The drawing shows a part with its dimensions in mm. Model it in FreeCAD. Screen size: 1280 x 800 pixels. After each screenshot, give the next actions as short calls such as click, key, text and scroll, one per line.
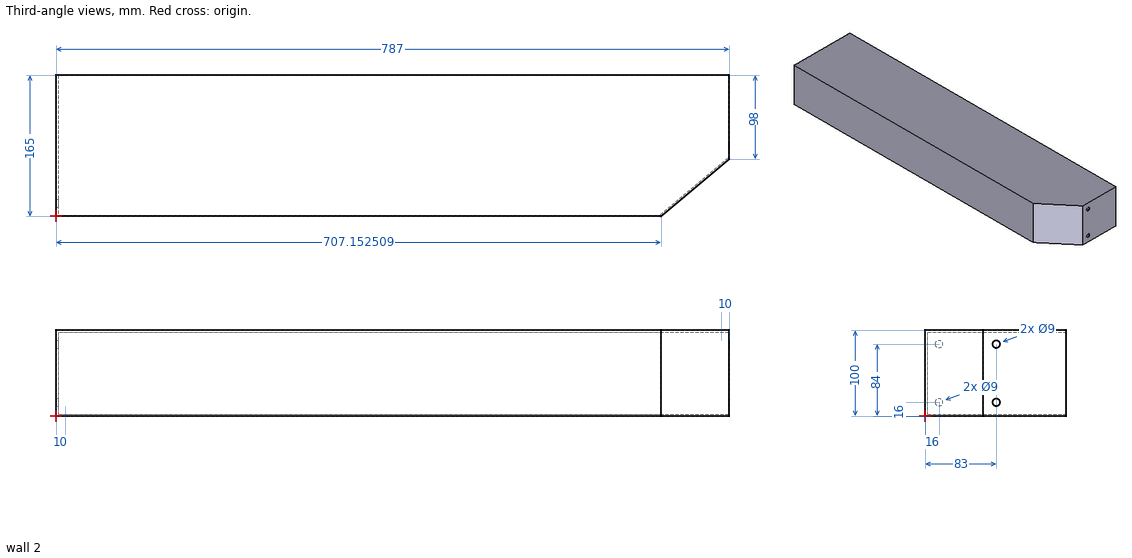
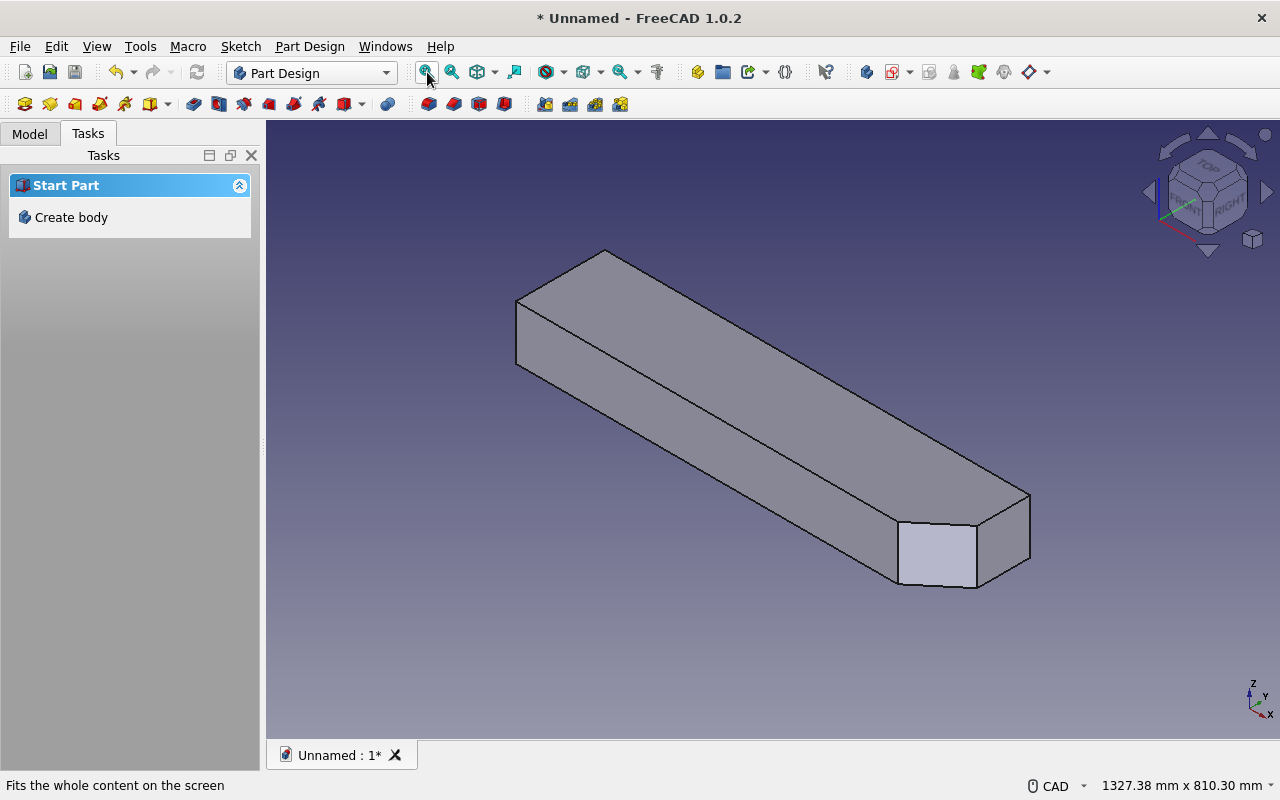
key(2)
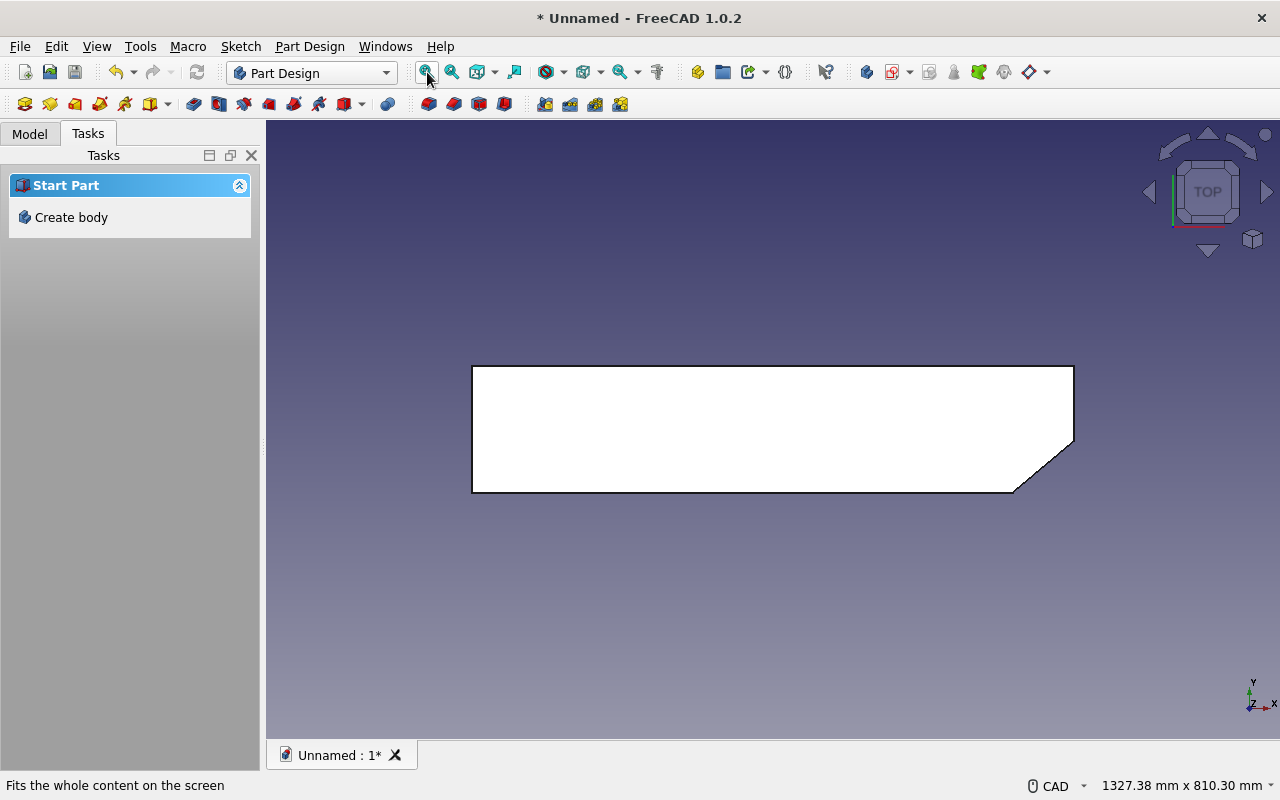
key(1)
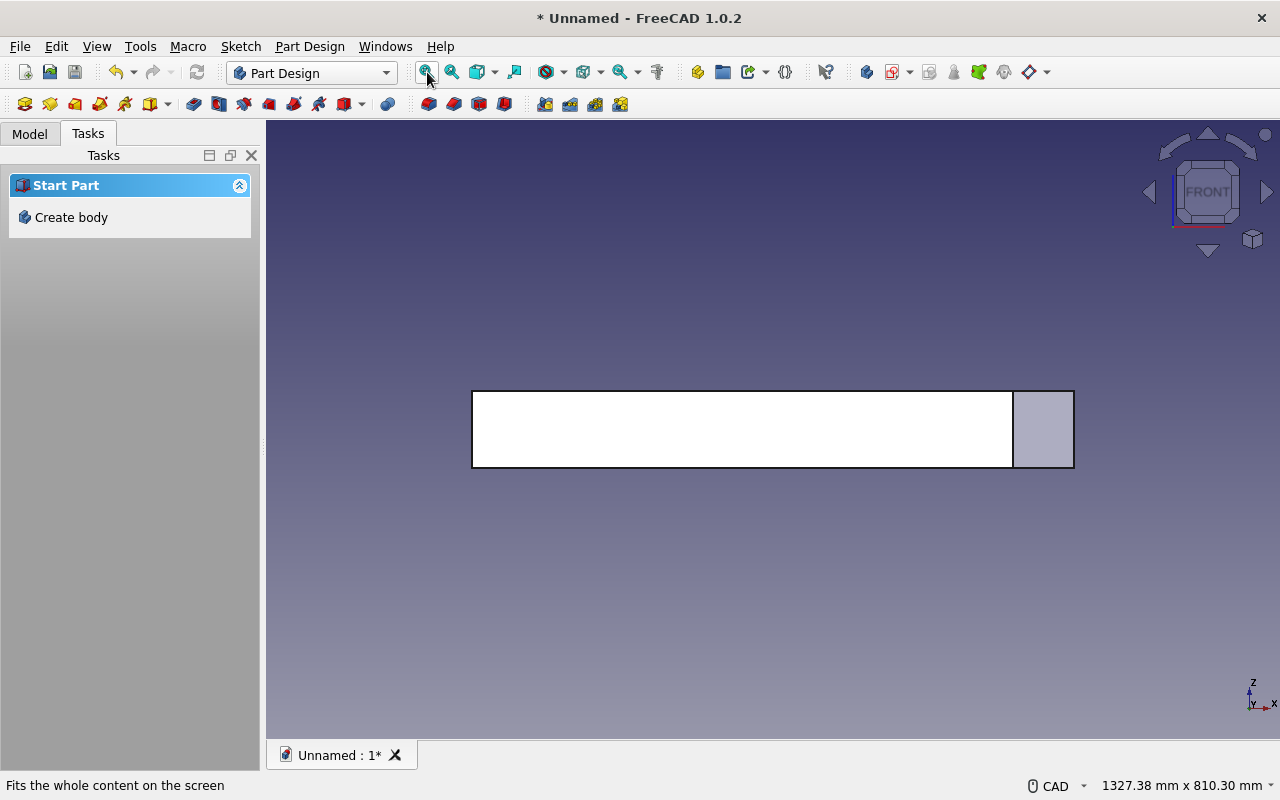
key(3)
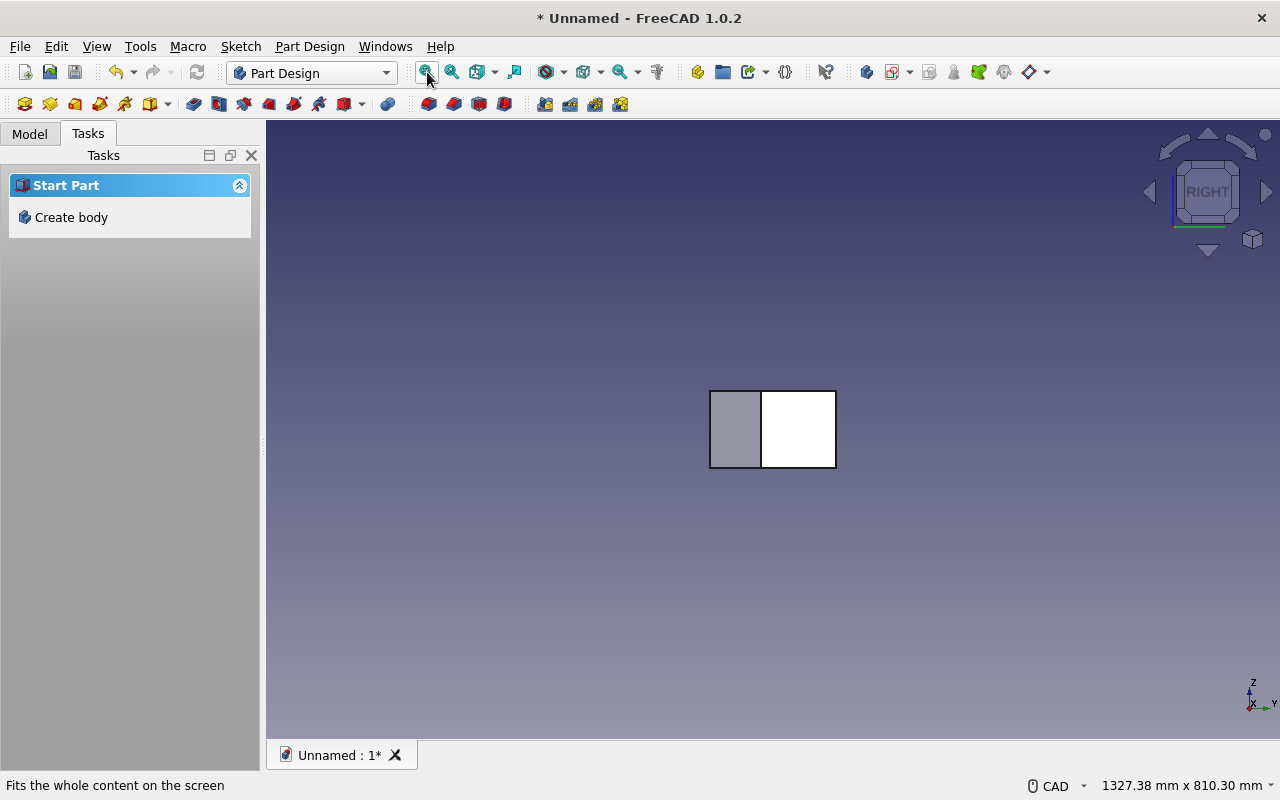
click(427, 72)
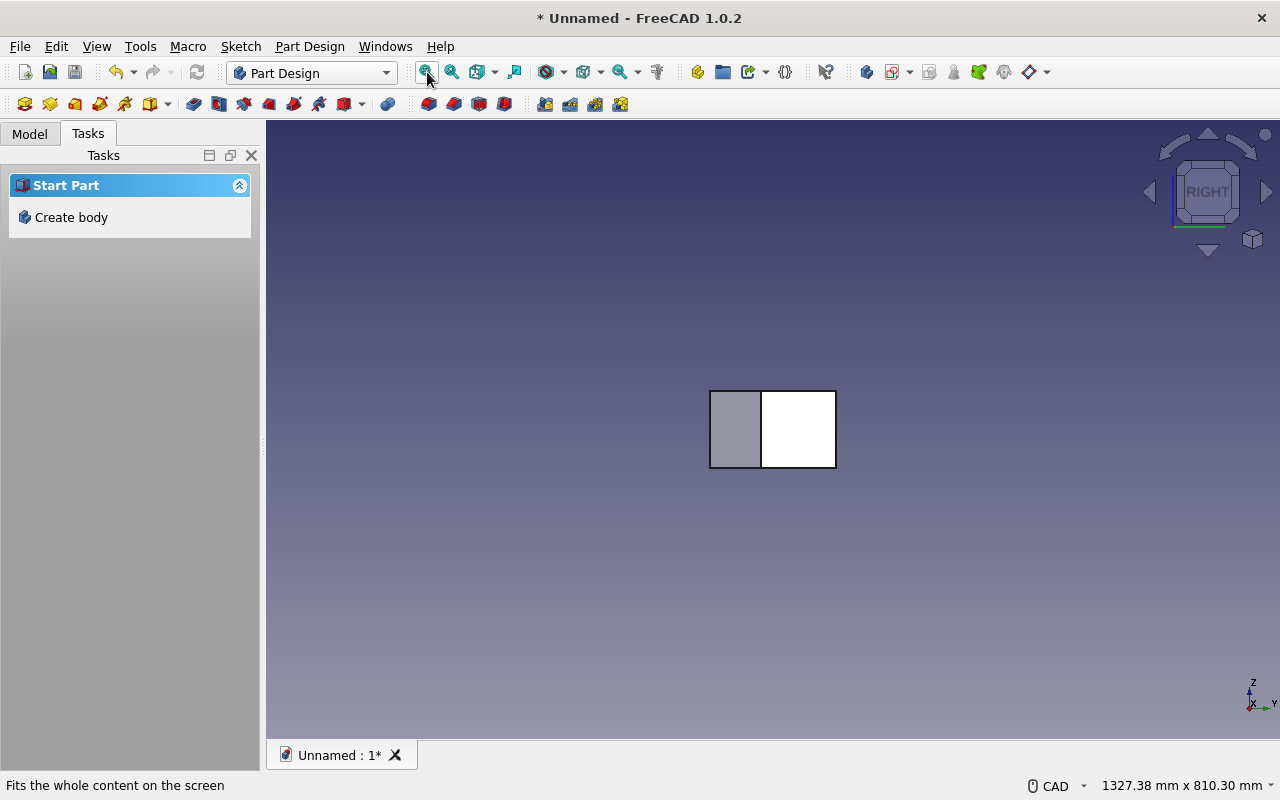
key(5)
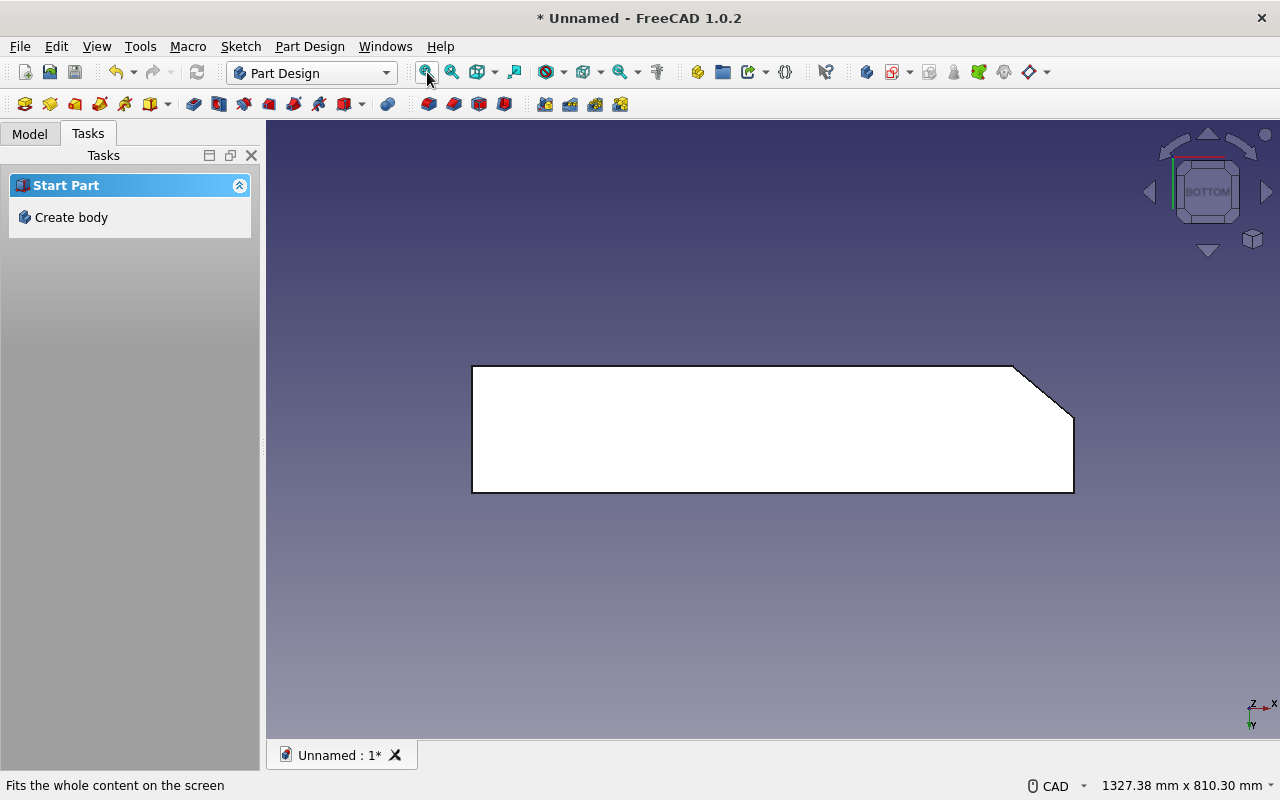
key(4)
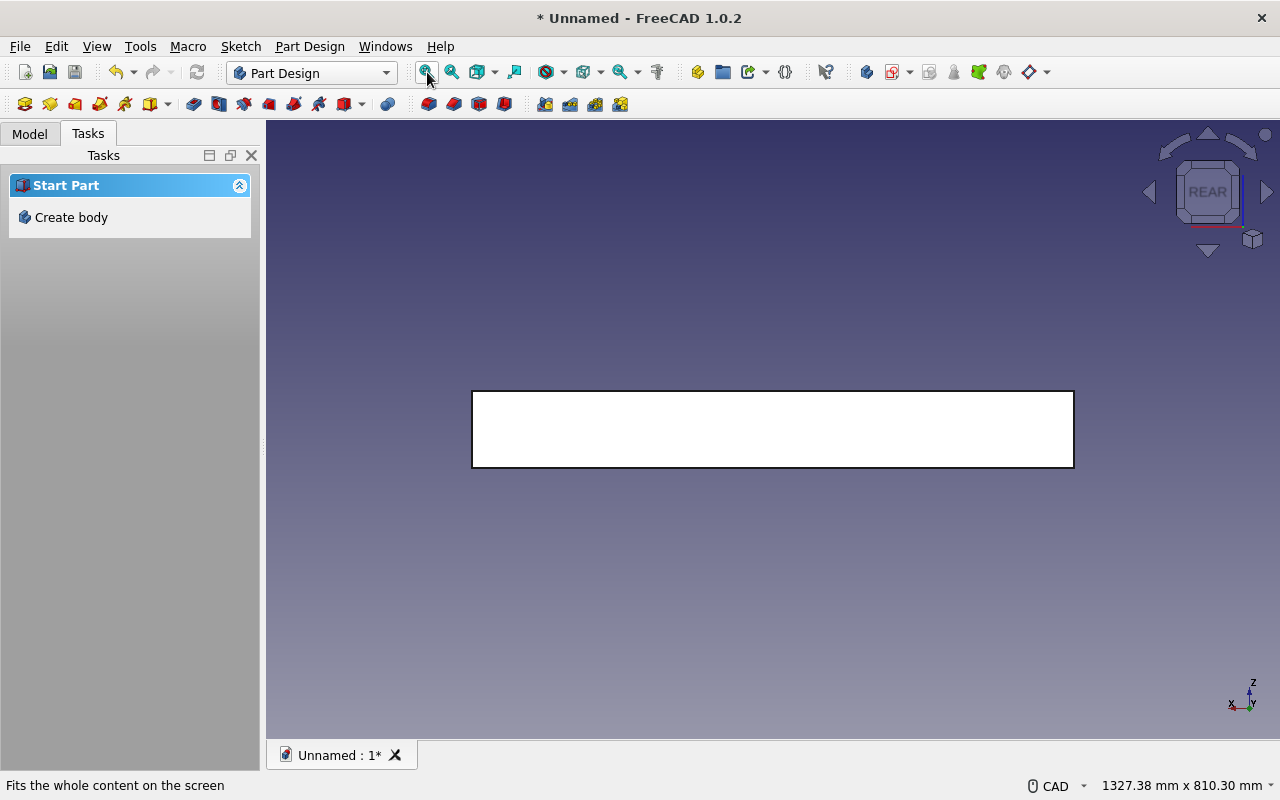
click(515, 429)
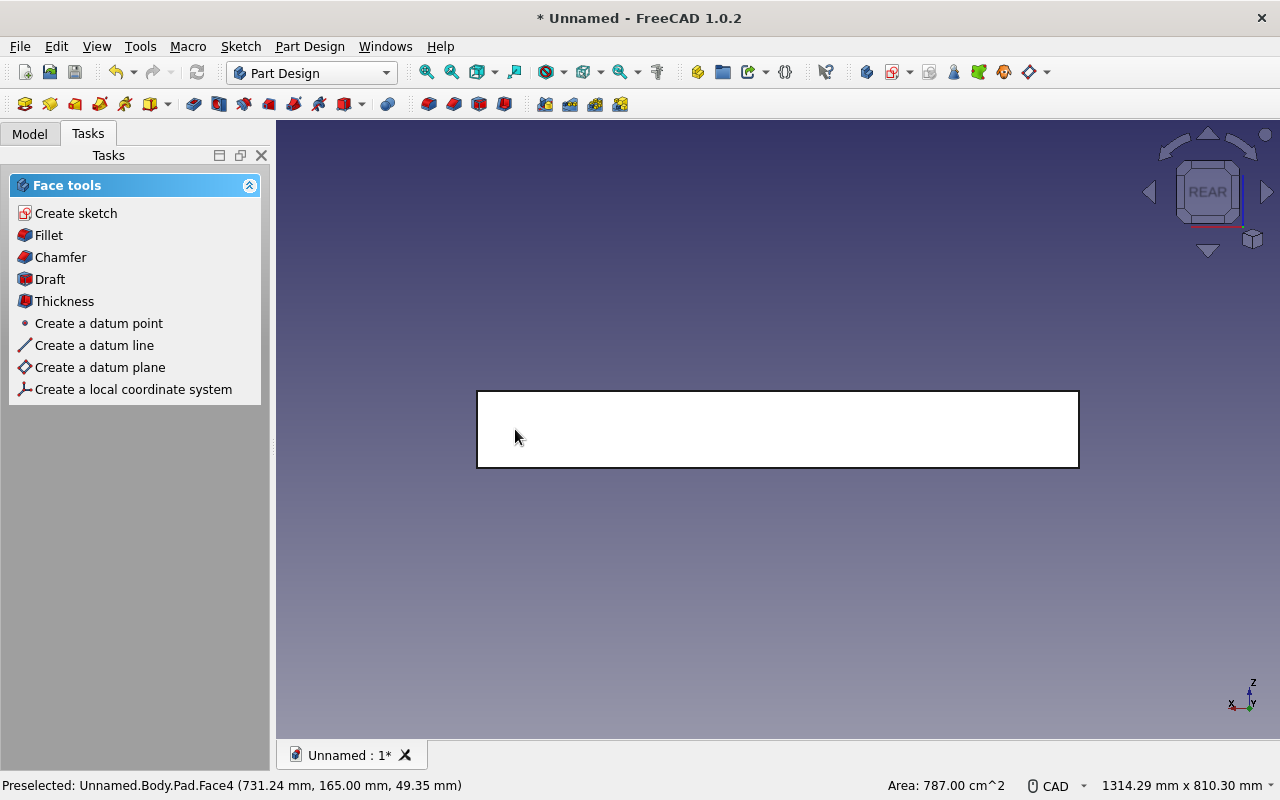
click(504, 104)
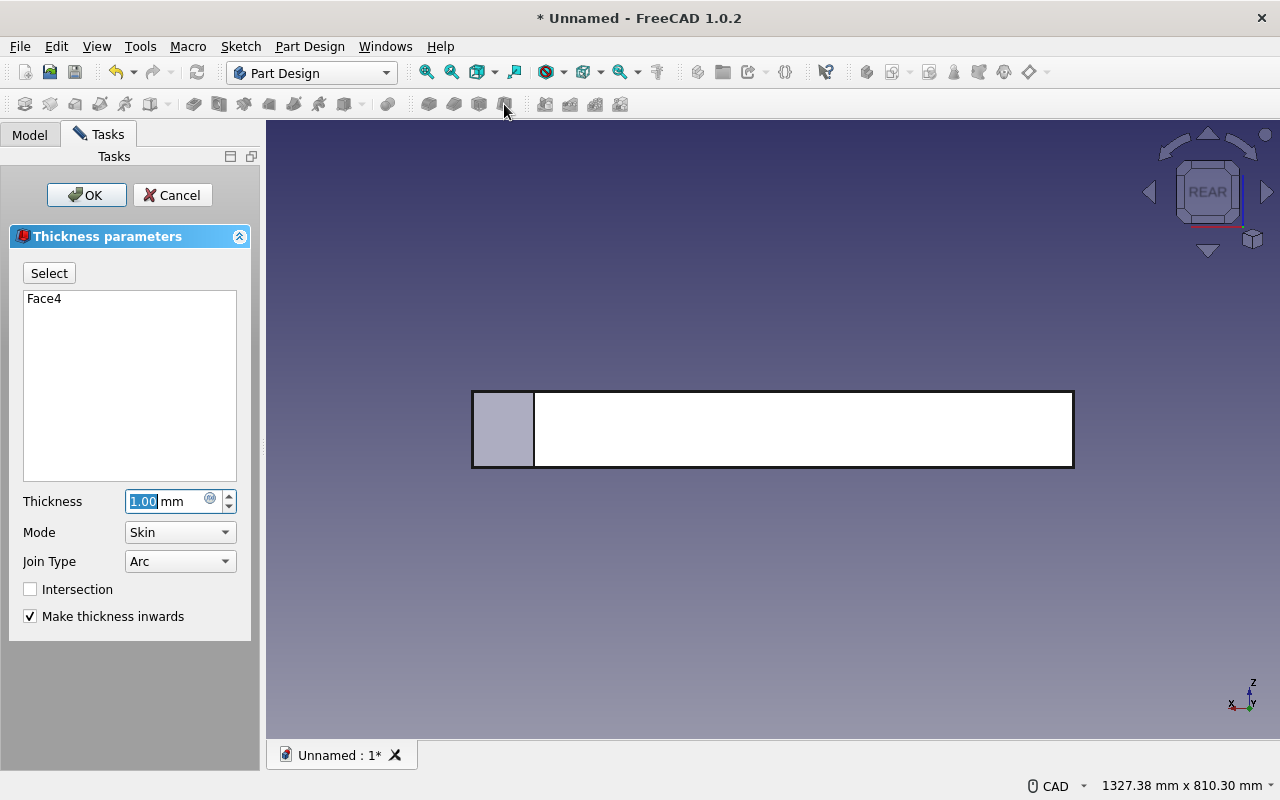
text(2)
key(Tab)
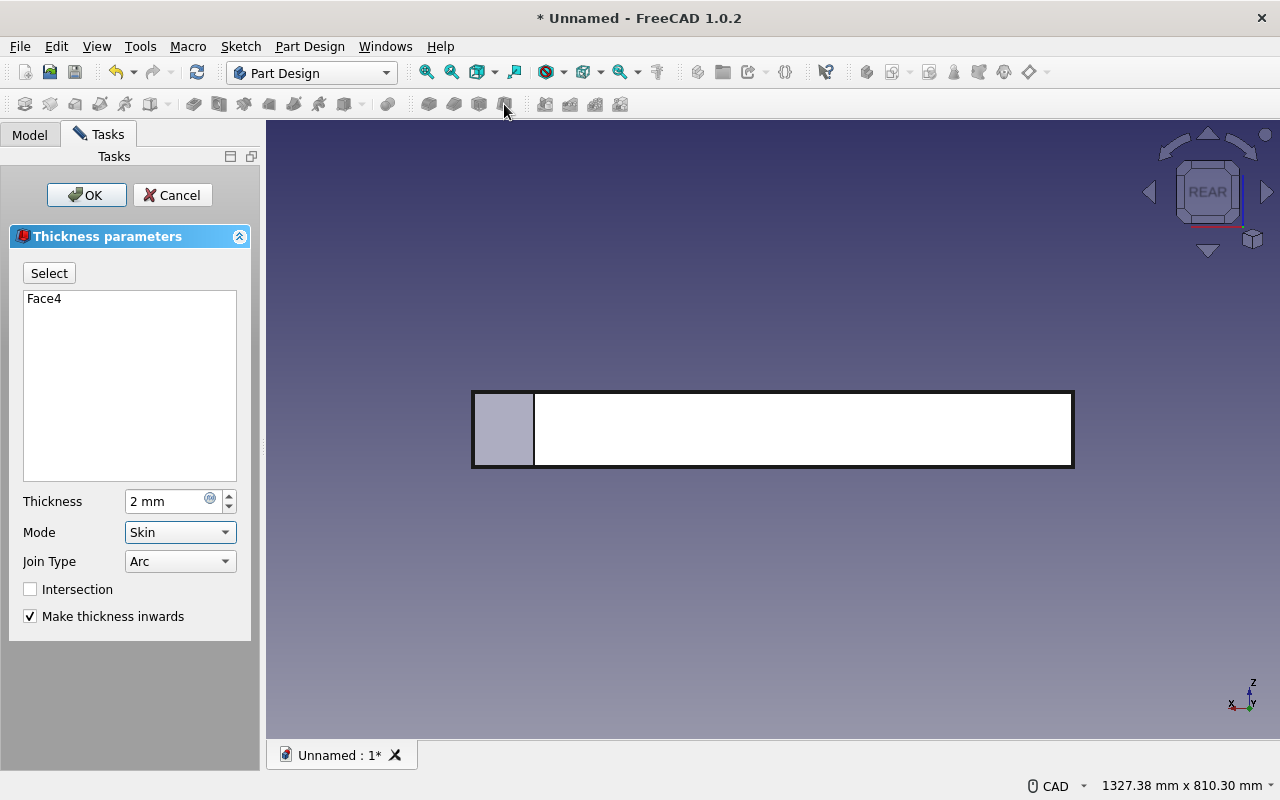
click(181, 562)